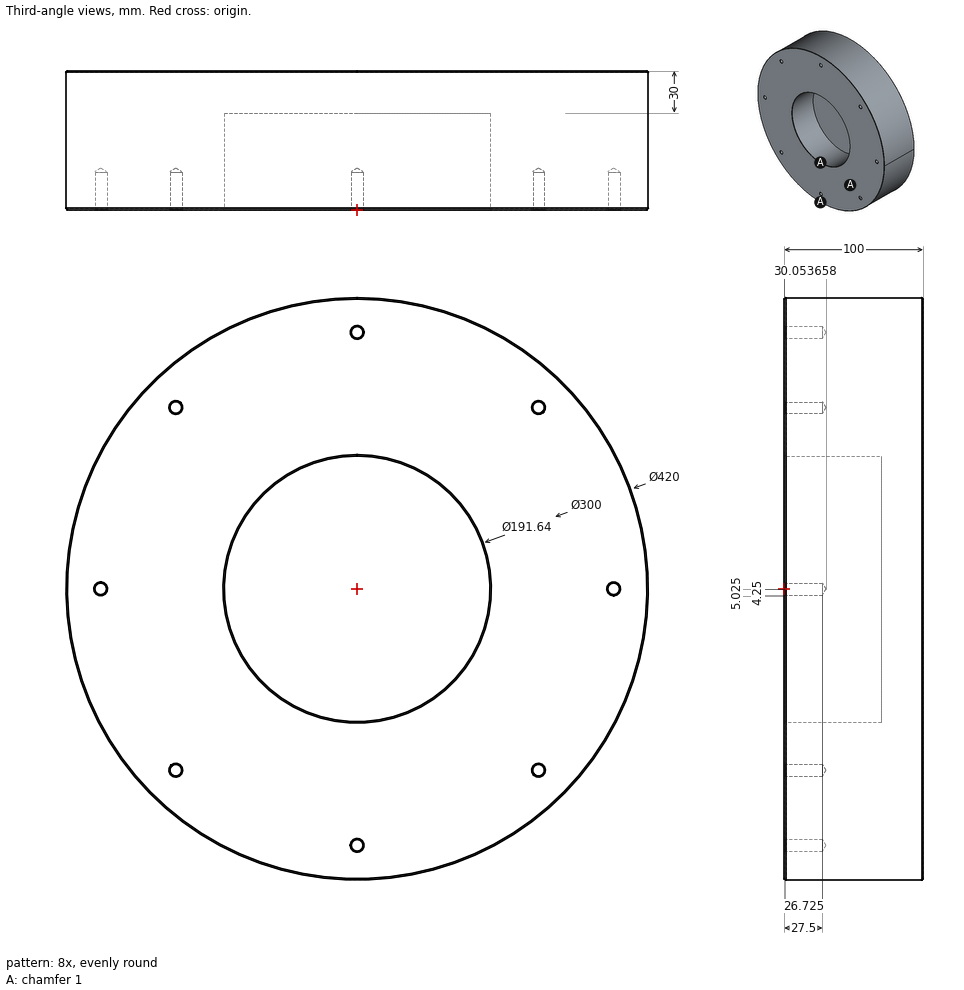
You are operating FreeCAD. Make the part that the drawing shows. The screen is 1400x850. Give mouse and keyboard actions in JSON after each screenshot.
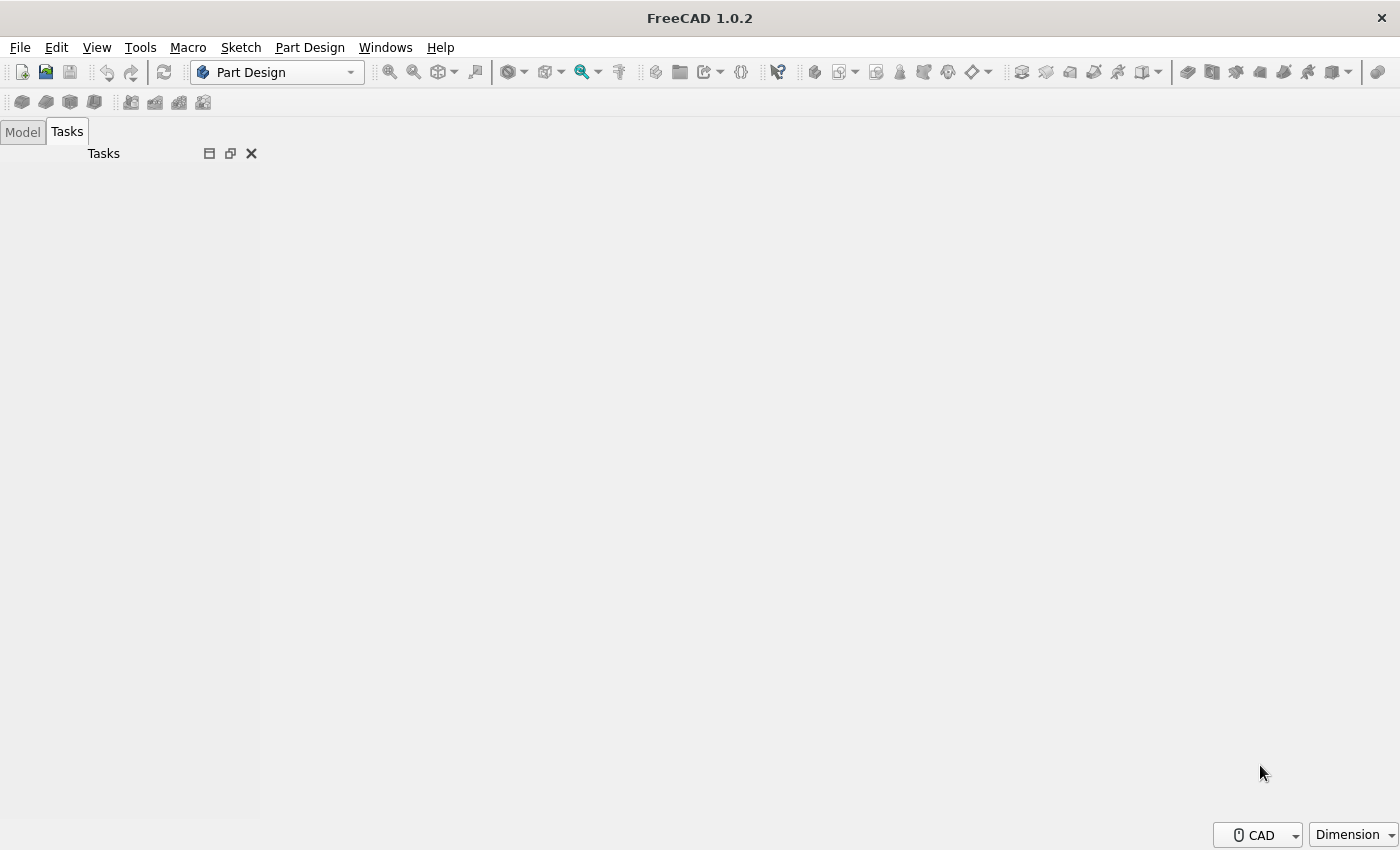
{"action": "key", "text": "ctrl+n"}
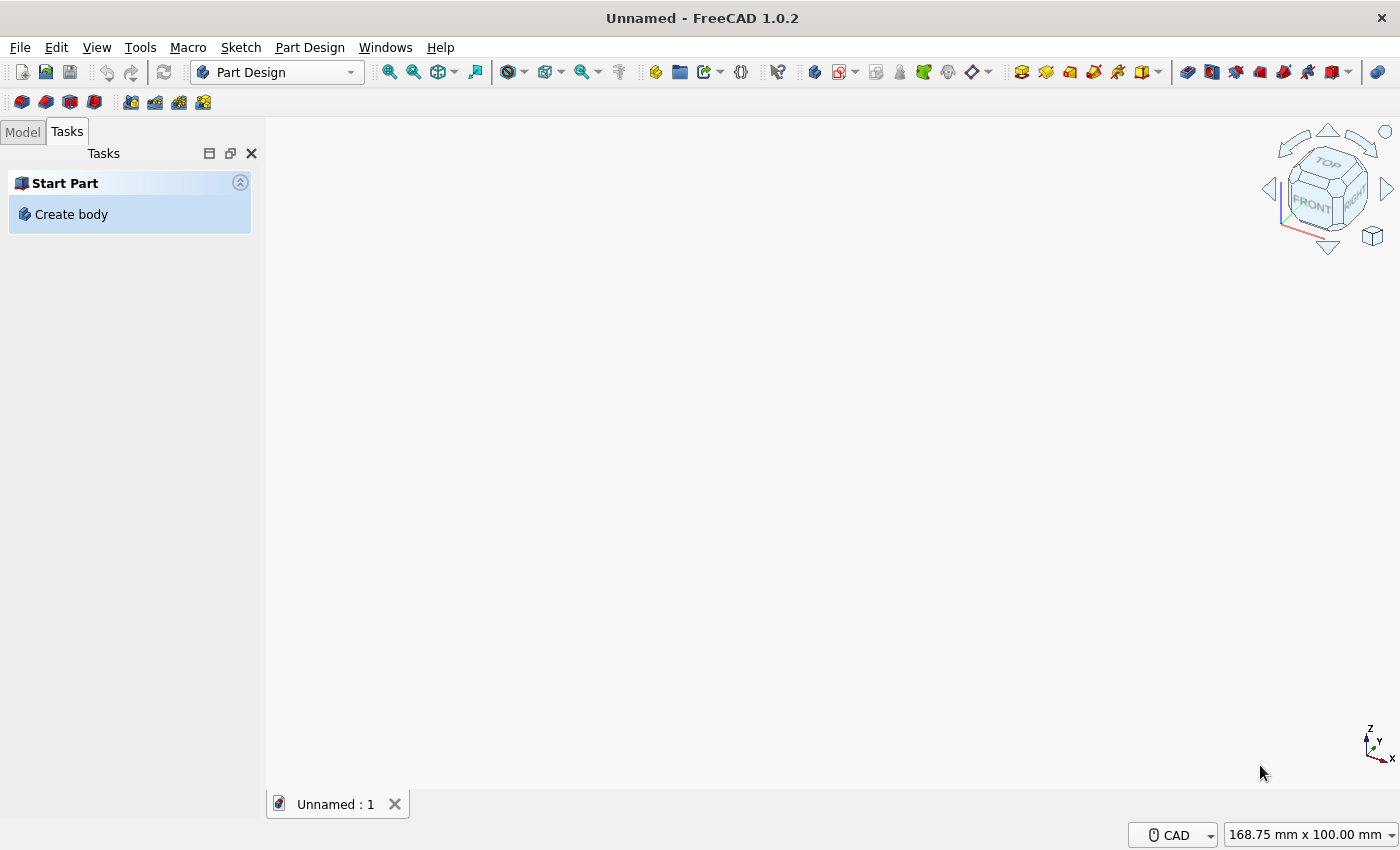
{"action": "left_click", "coordinate": [840, 72]}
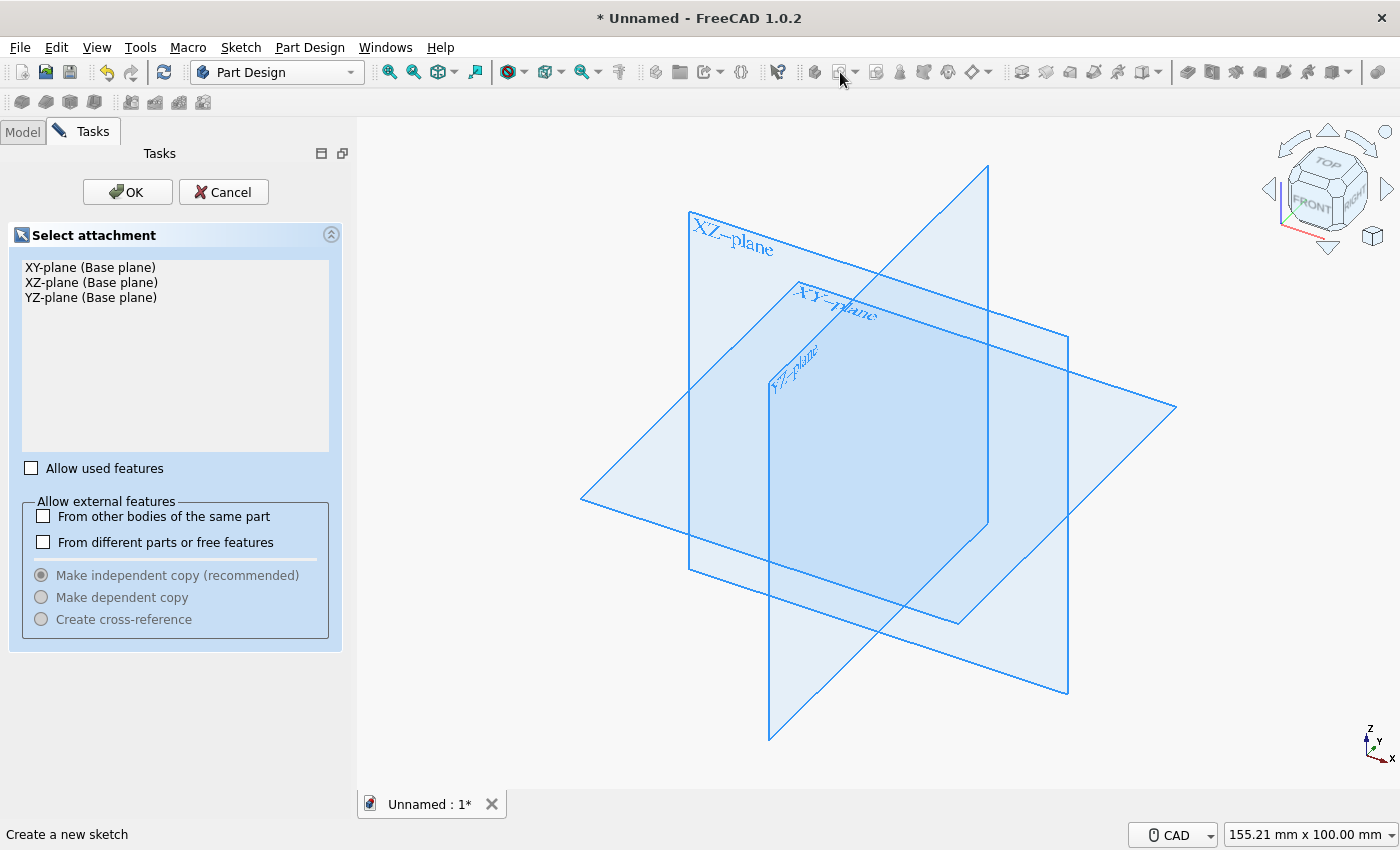
{"action": "left_click", "coordinate": [82, 282]}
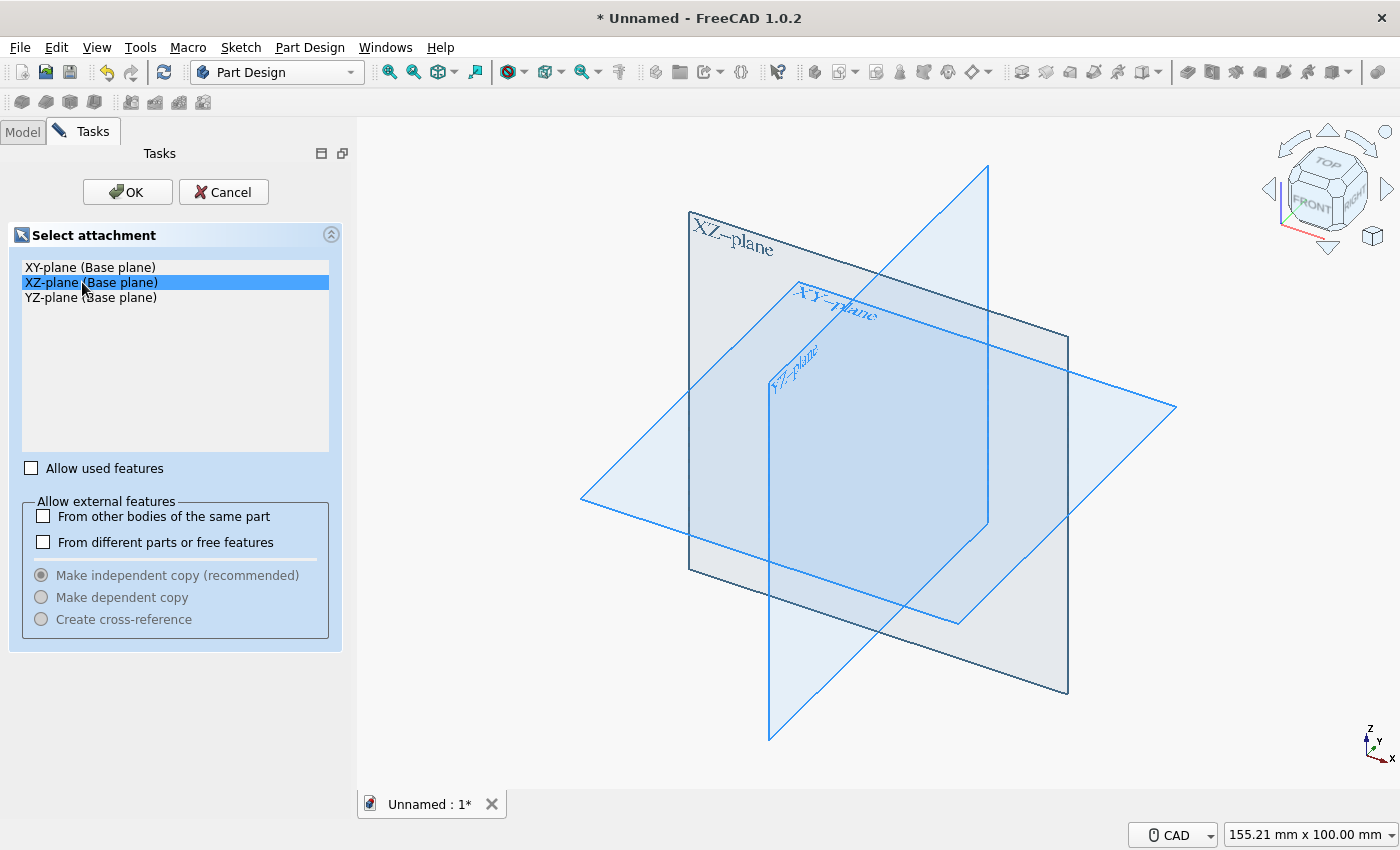
{"action": "left_click", "coordinate": [128, 192]}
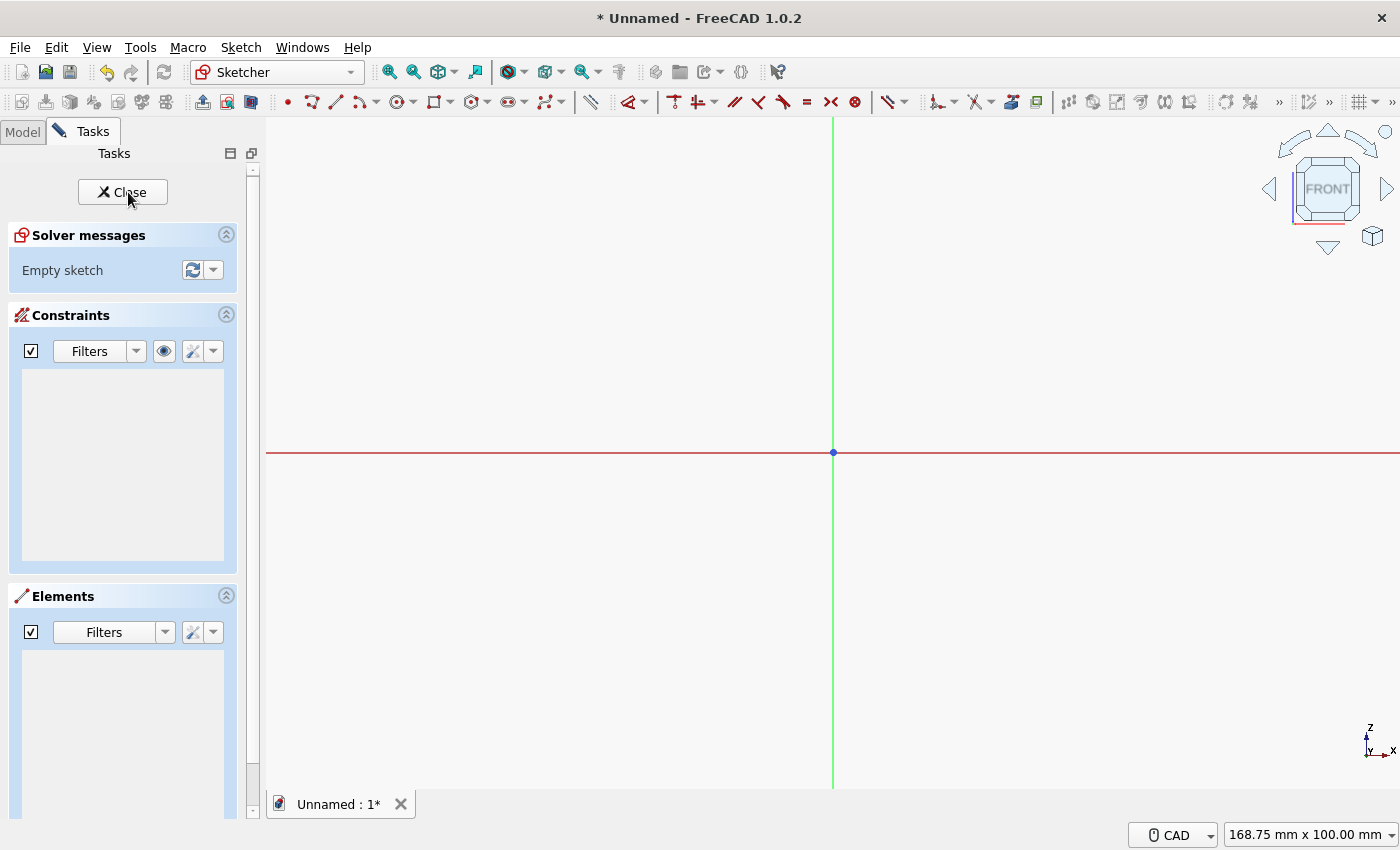
{"action": "scroll", "coordinate": [751, 453], "scroll_direction": "down", "scroll_amount": 9}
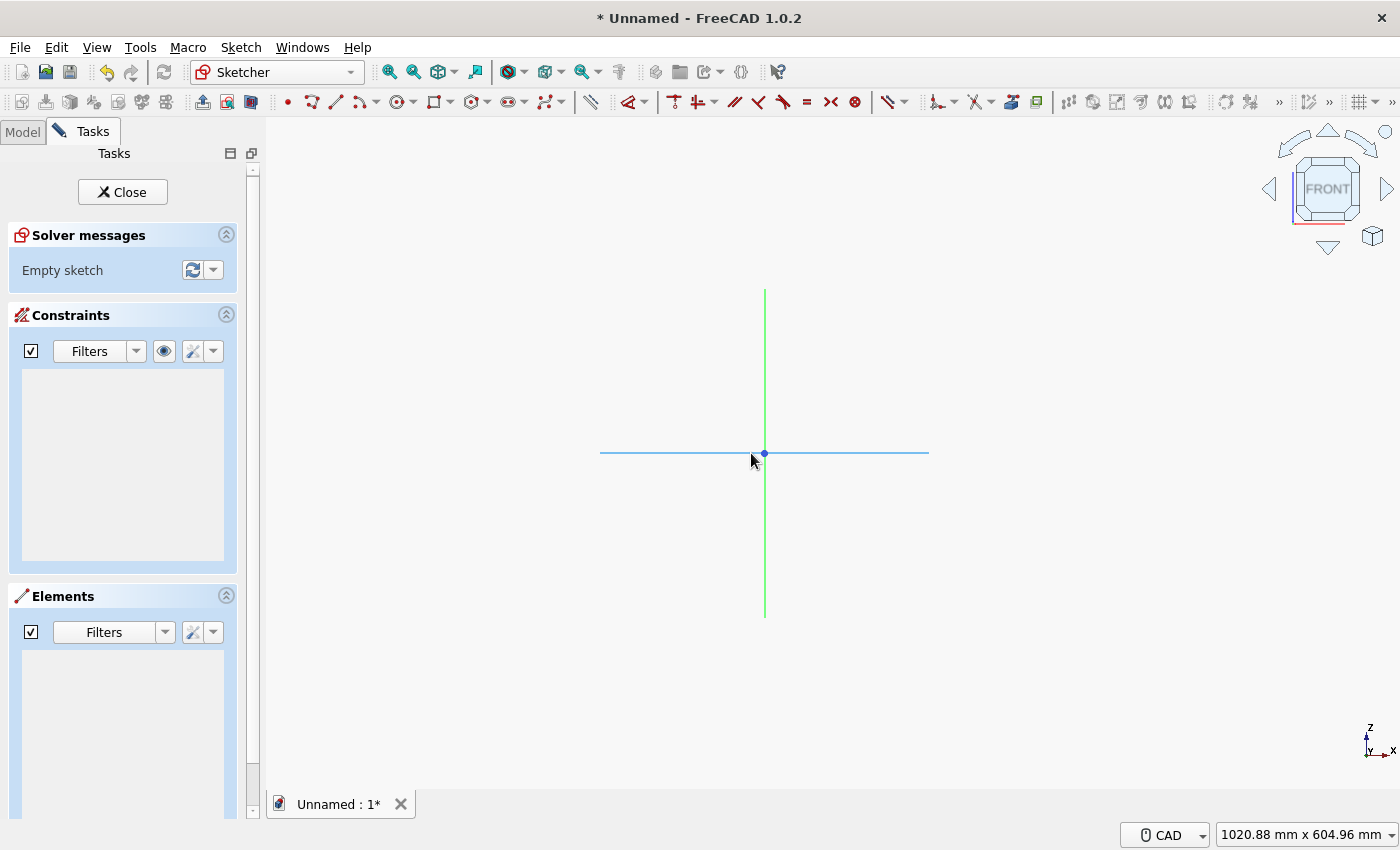
{"action": "key", "text": "g c"}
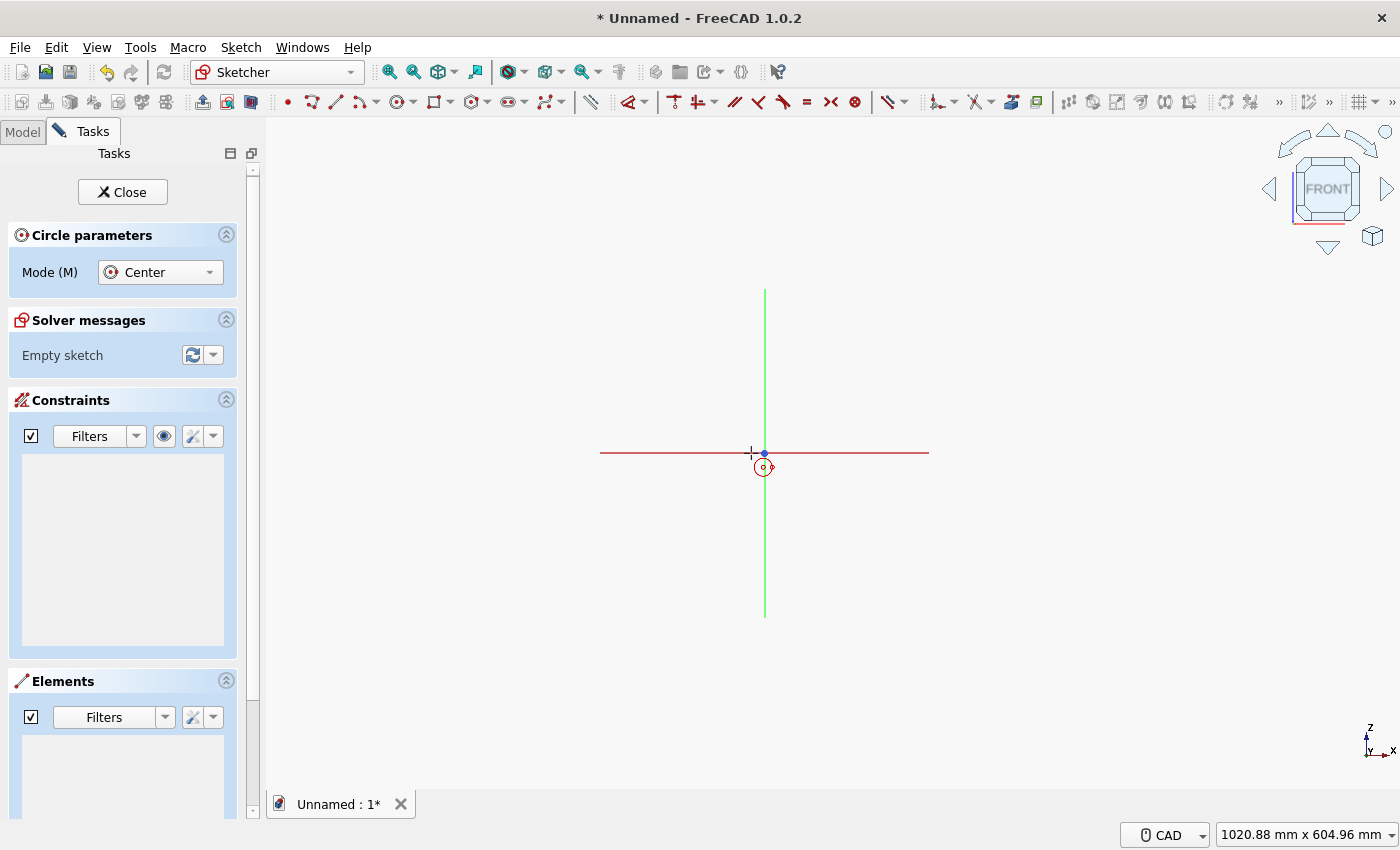
{"action": "left_click", "coordinate": [765, 453]}
{"action": "left_click", "coordinate": [930, 288]}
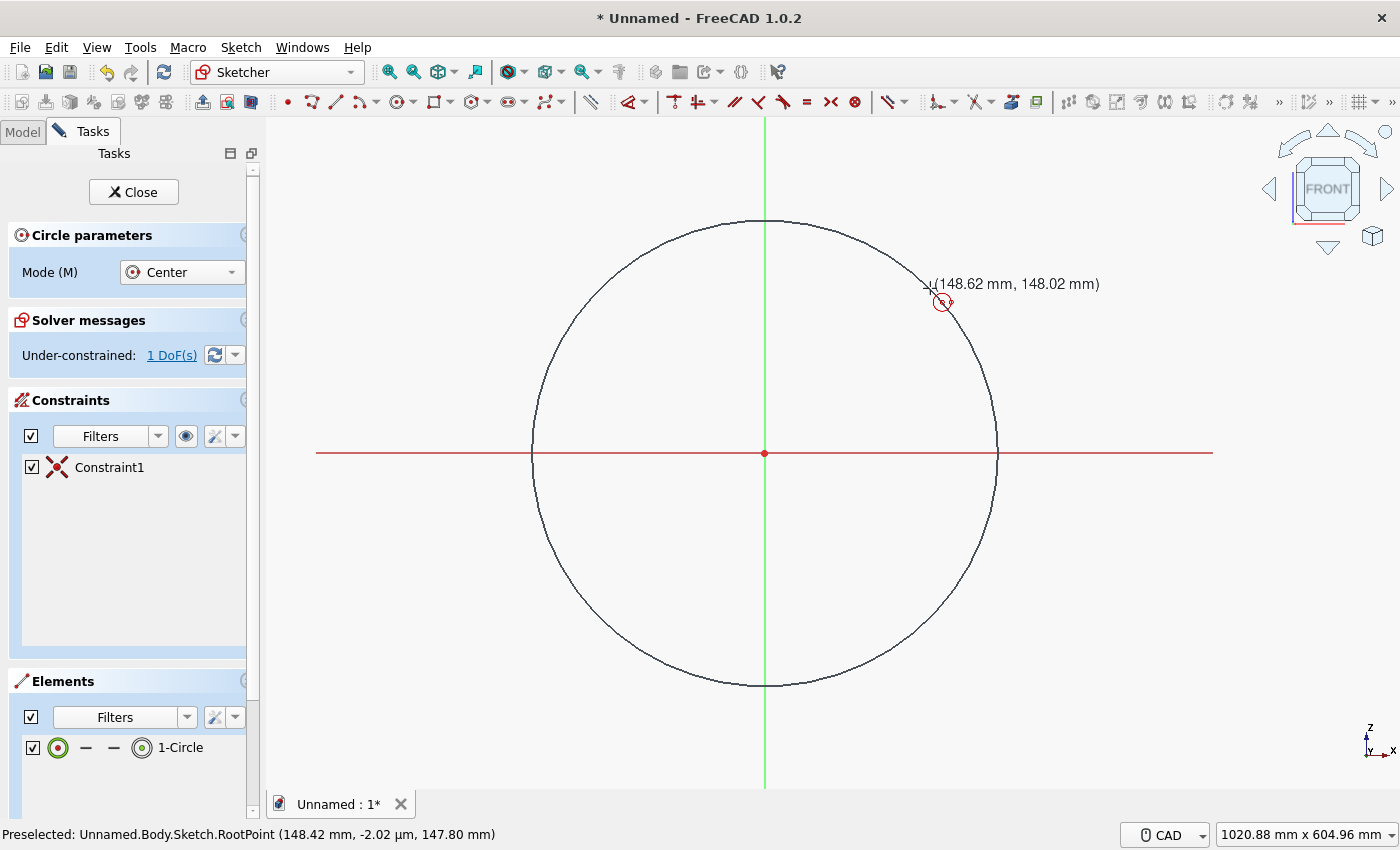
{"action": "left_click", "coordinate": [765, 453]}
{"action": "left_click", "coordinate": [840, 378]}
{"action": "key", "text": "Escape"}